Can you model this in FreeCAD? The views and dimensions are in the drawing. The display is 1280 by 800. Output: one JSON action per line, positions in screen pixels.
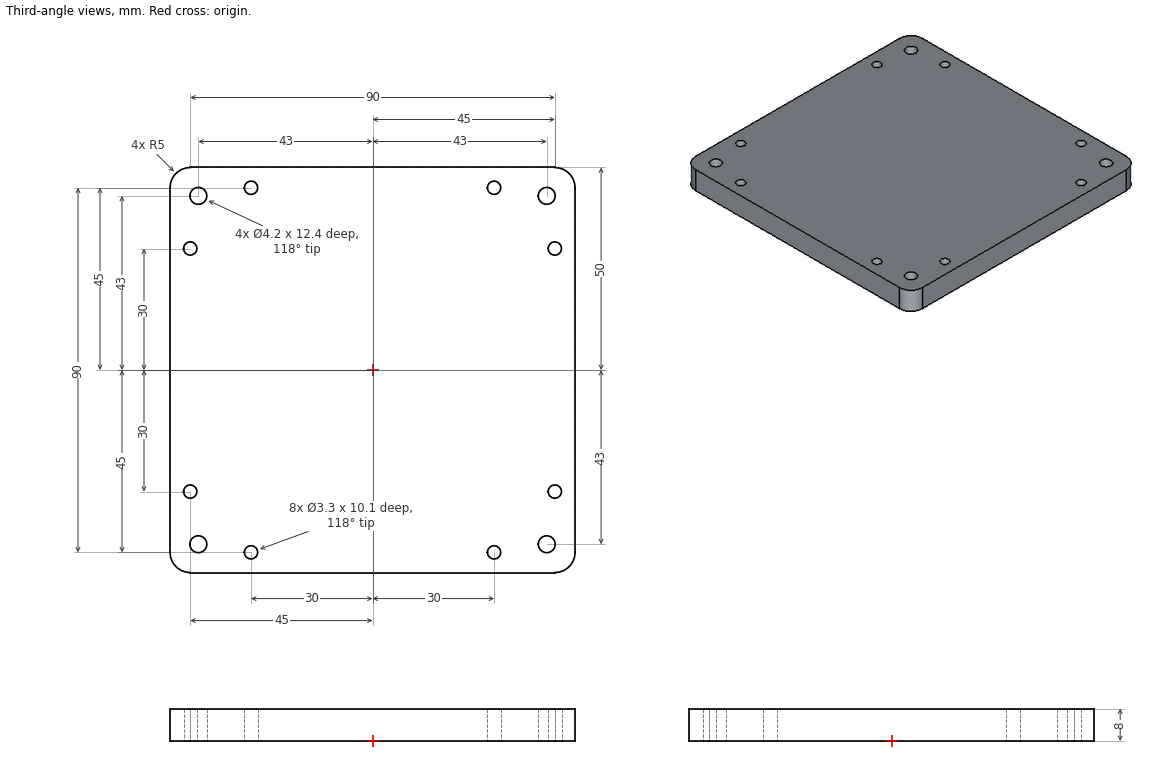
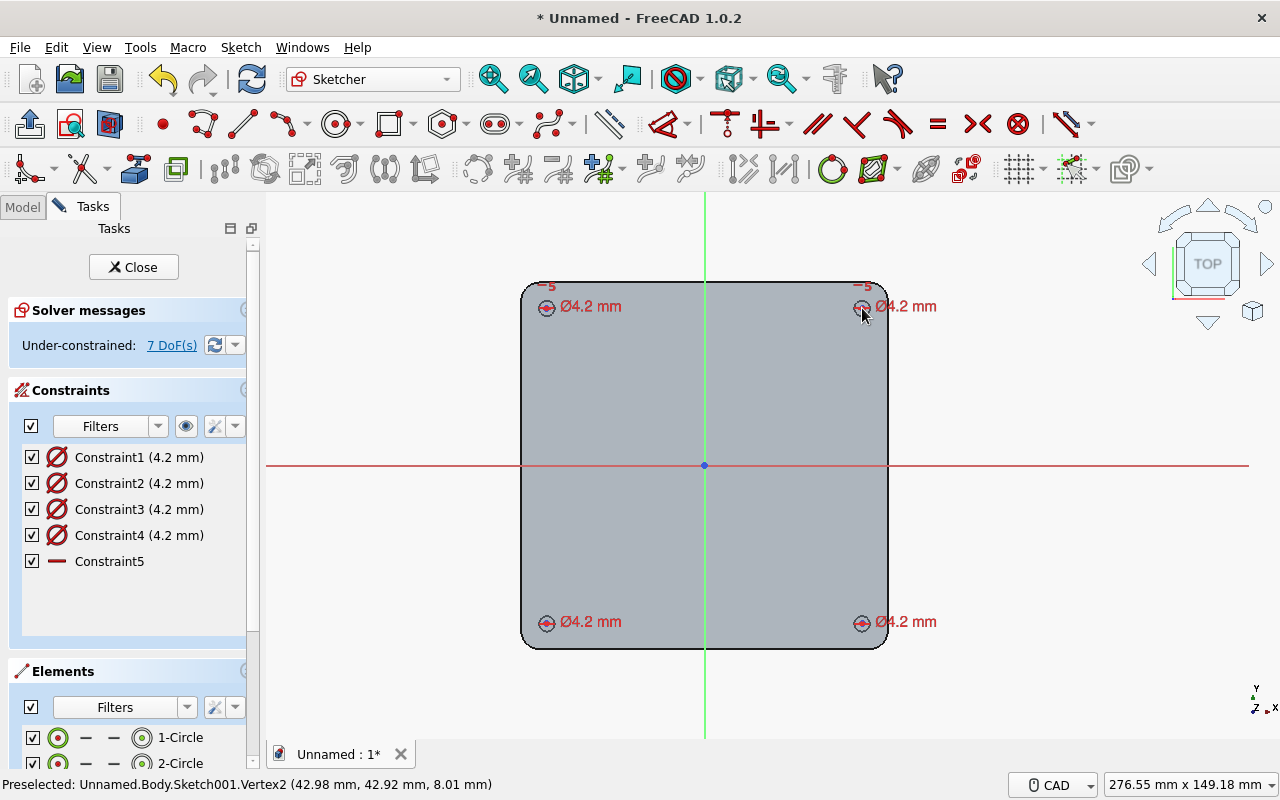
{"action": "left_click", "coordinate": [862, 308]}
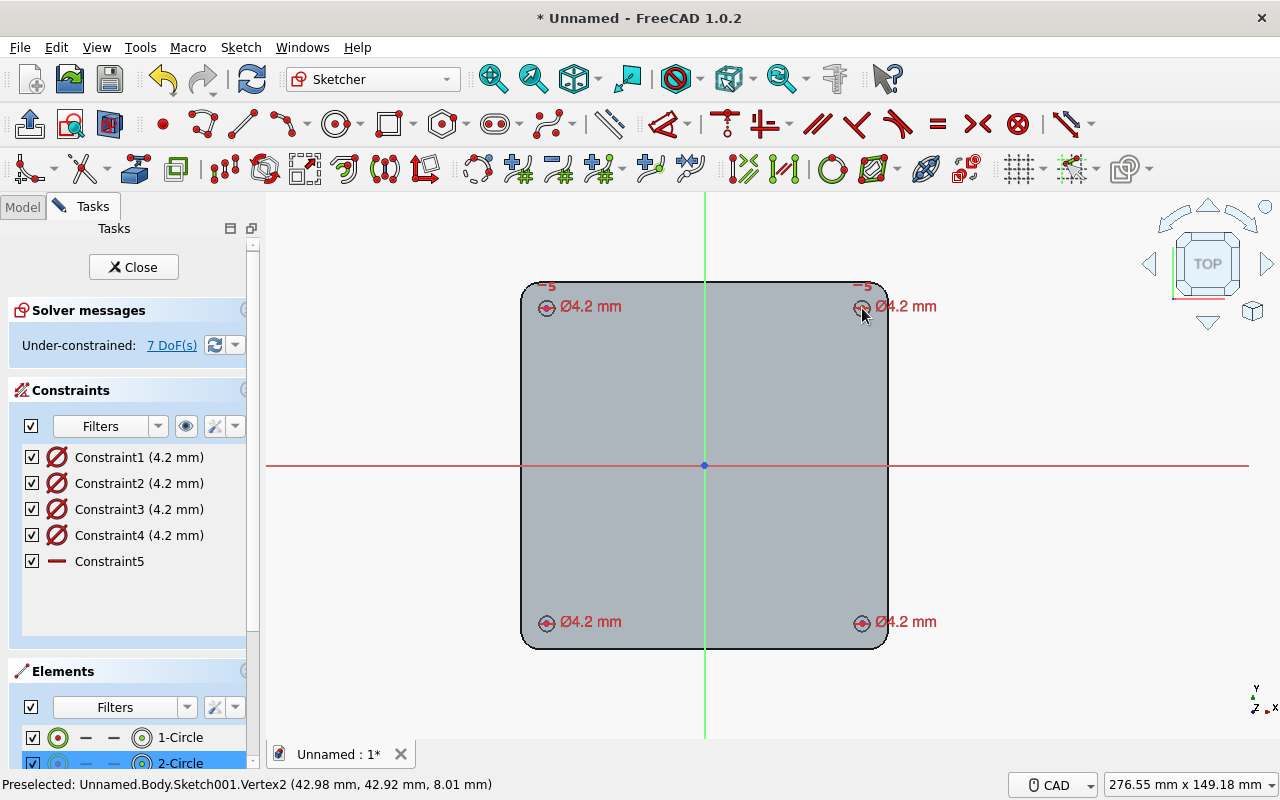
{"action": "left_click", "coordinate": [862, 624]}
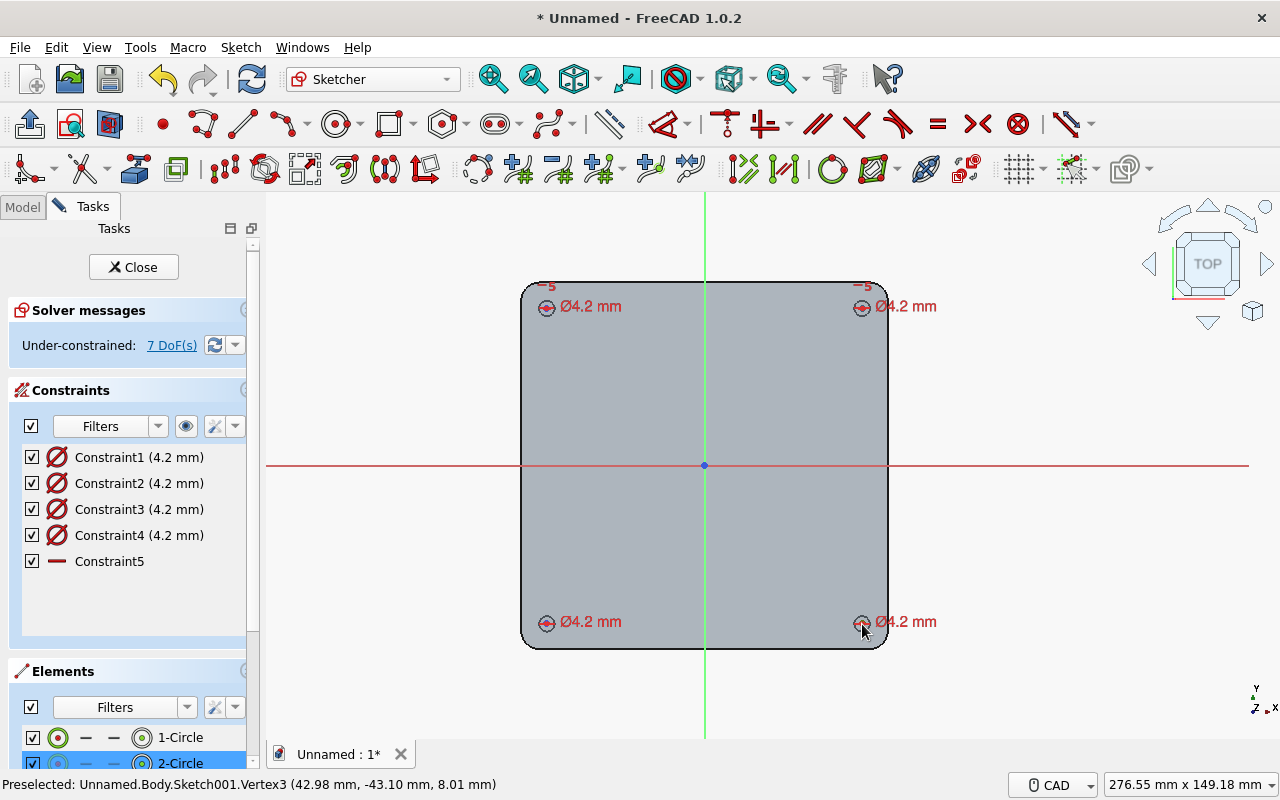
{"action": "key", "text": "v"}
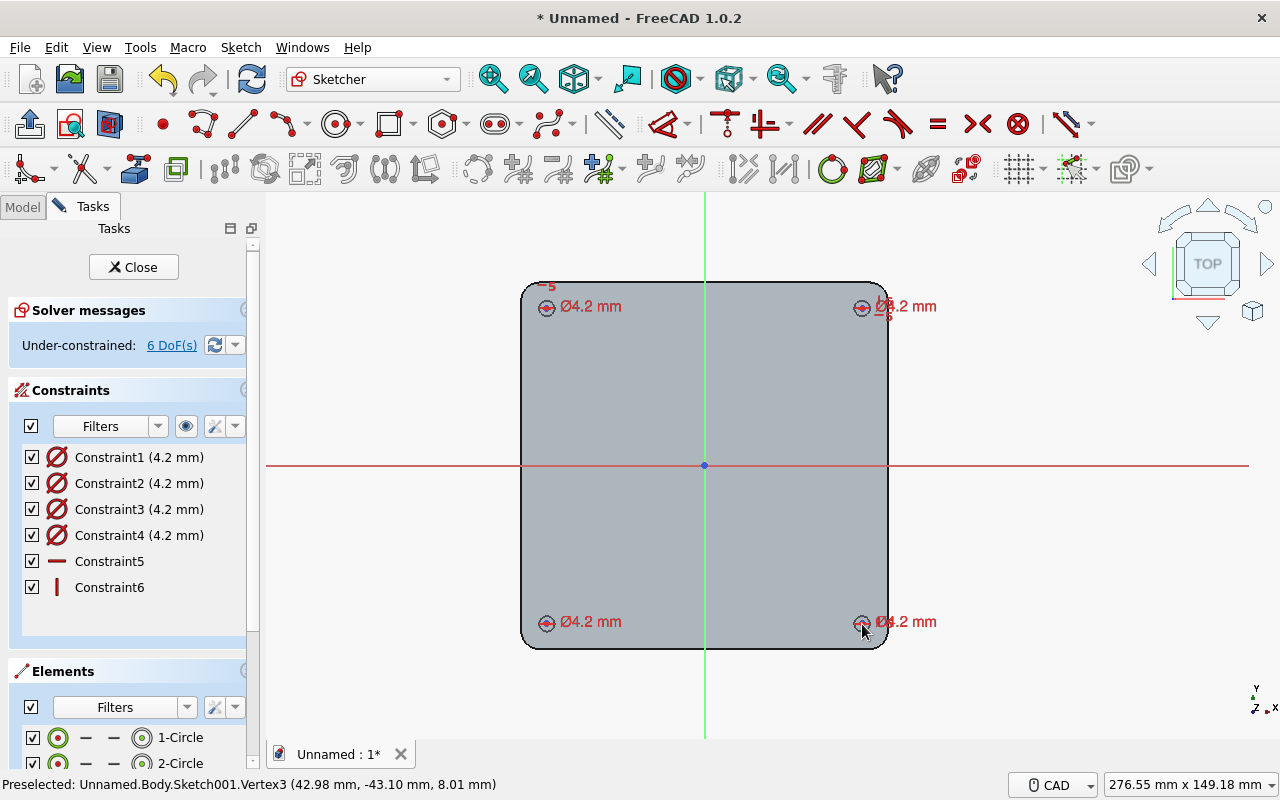
{"action": "left_click", "coordinate": [547, 308]}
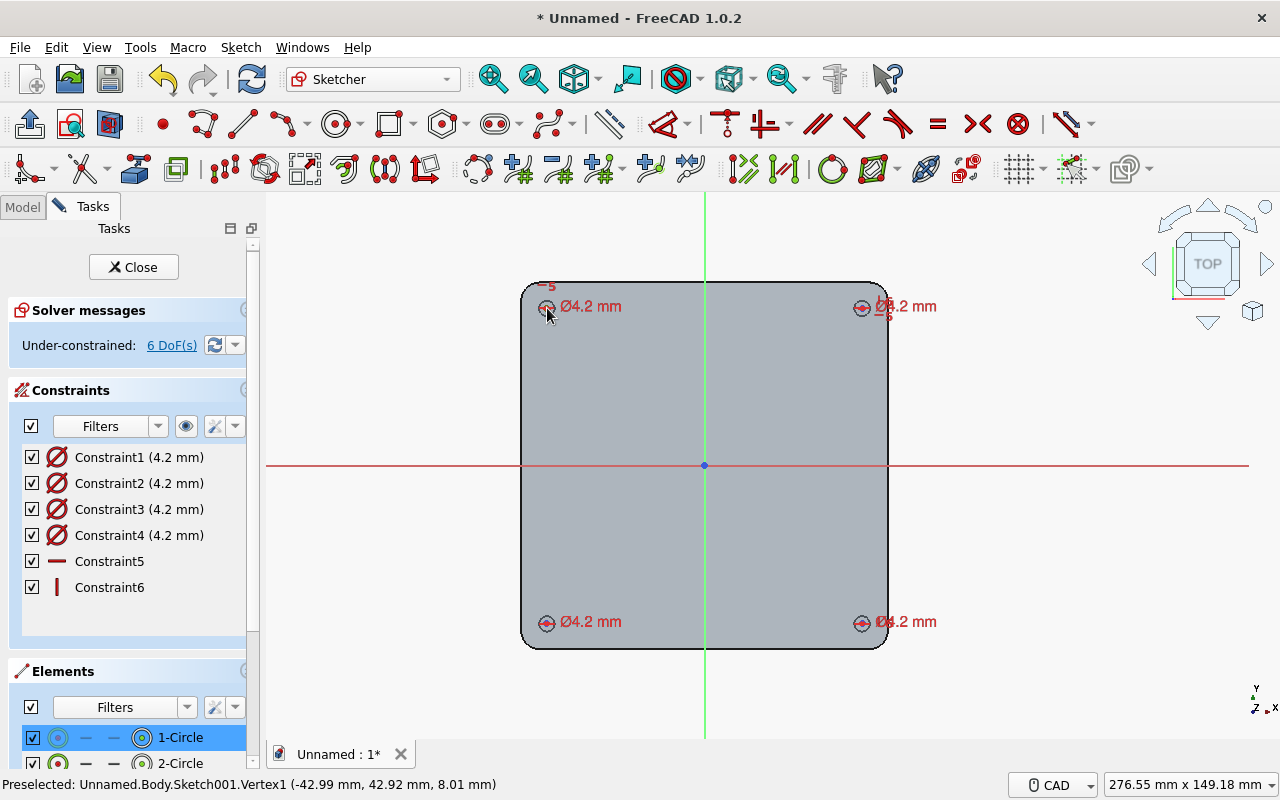
{"action": "left_click", "coordinate": [547, 624]}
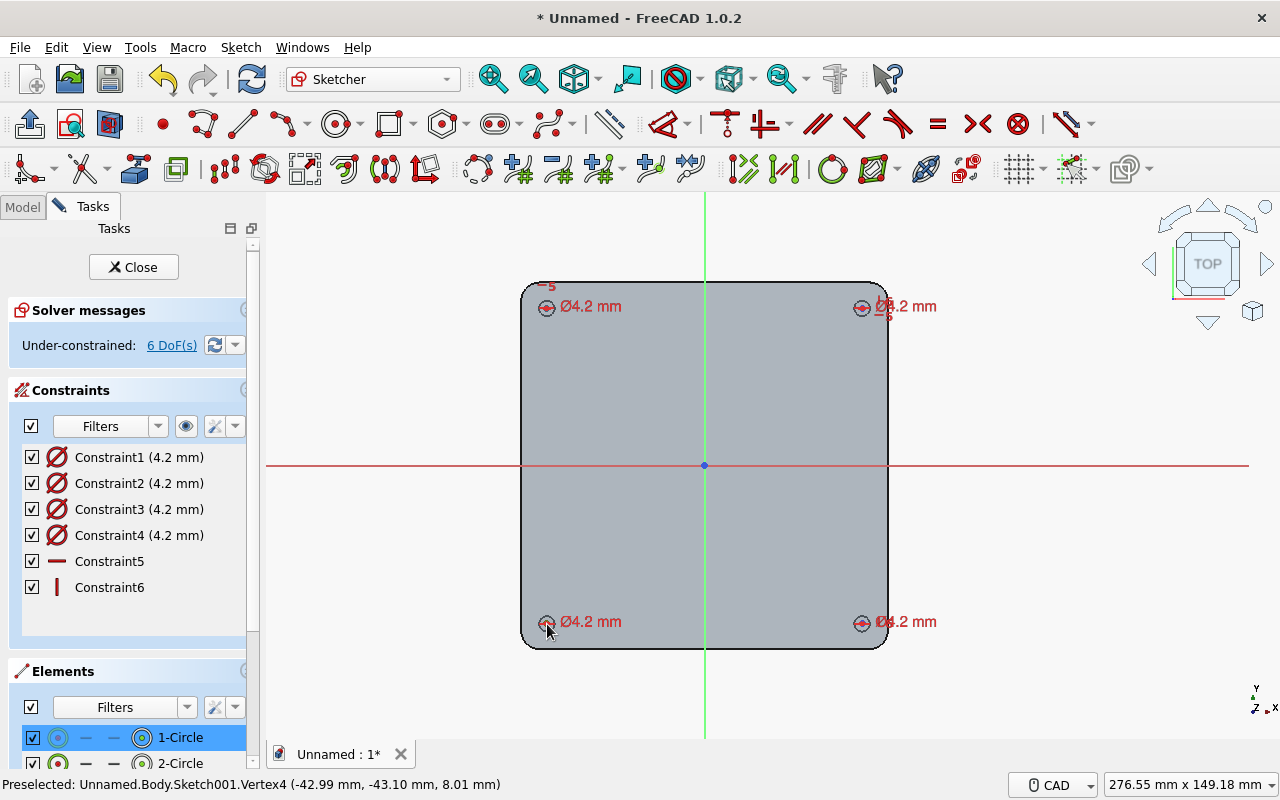
{"action": "key", "text": "v"}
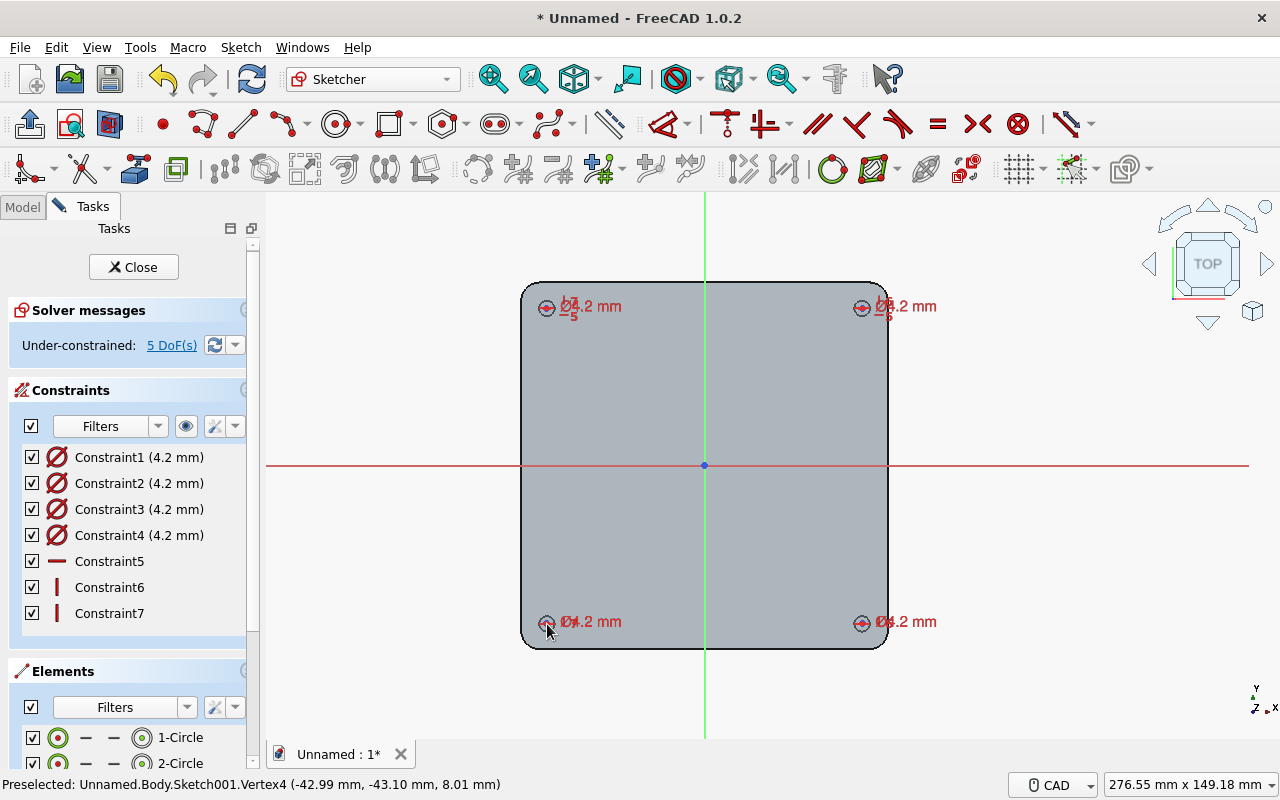
{"action": "left_click", "coordinate": [862, 624]}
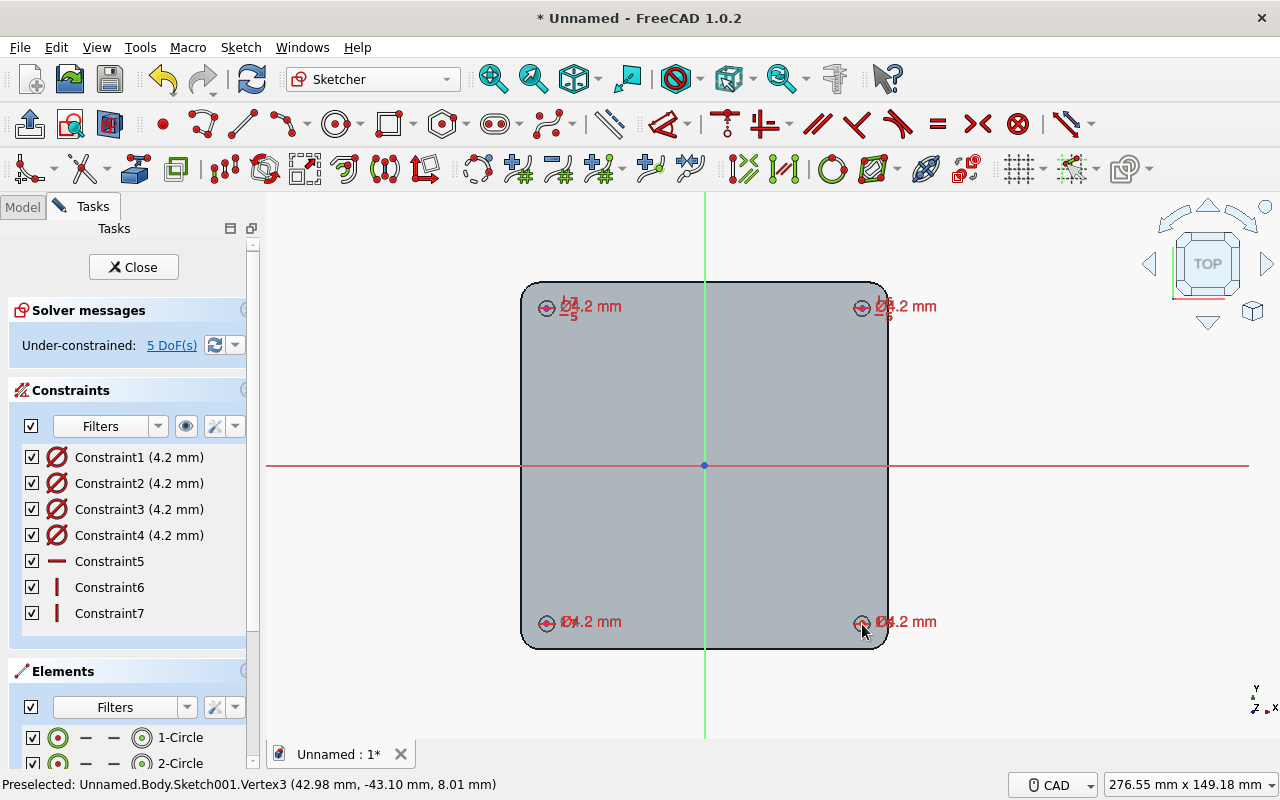
{"action": "left_click", "coordinate": [547, 624]}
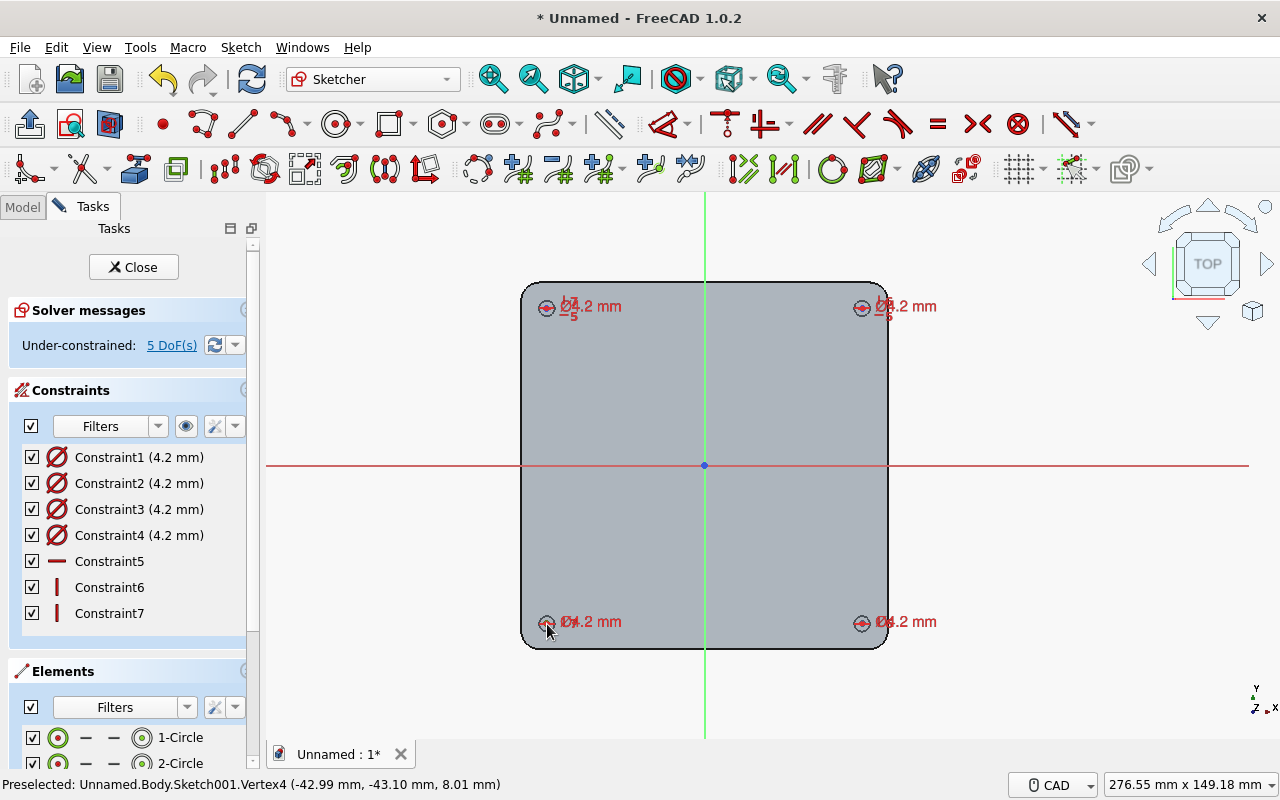
{"action": "key", "text": "h"}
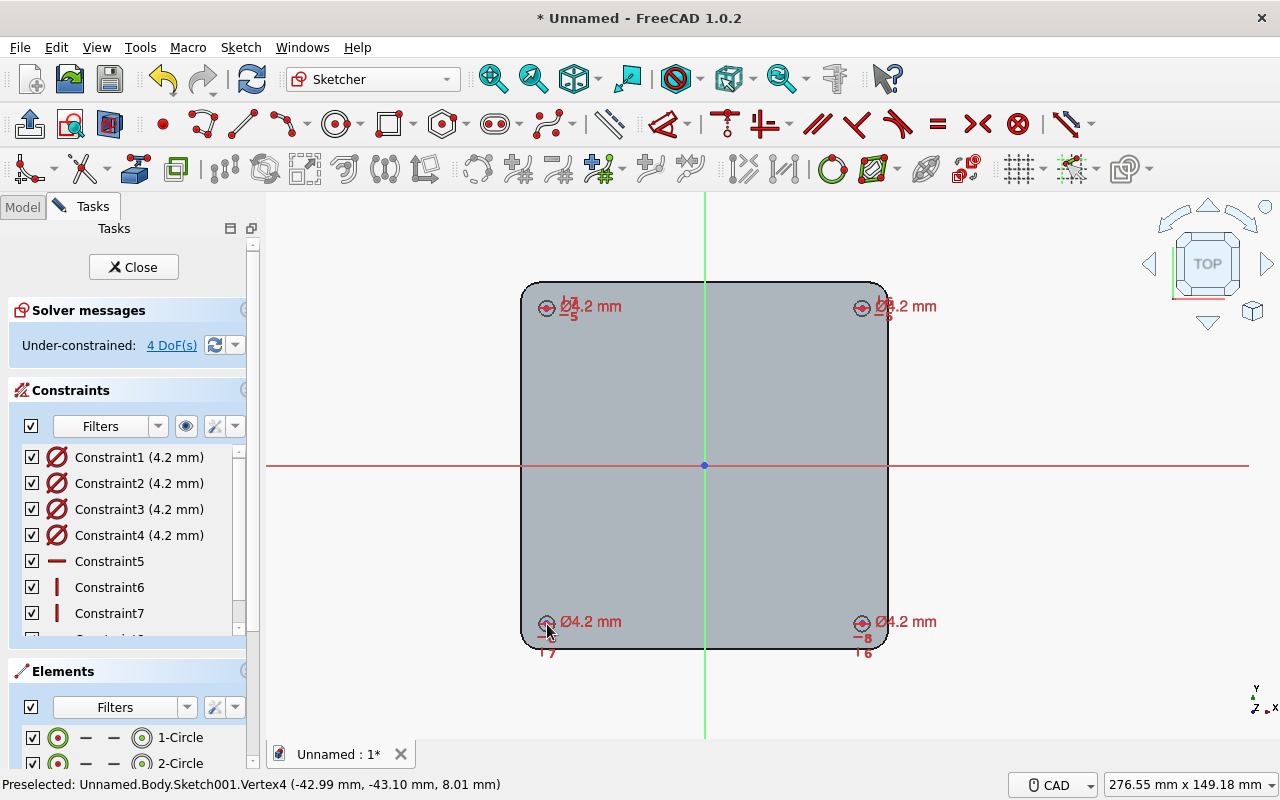
{"action": "left_click", "coordinate": [664, 124]}